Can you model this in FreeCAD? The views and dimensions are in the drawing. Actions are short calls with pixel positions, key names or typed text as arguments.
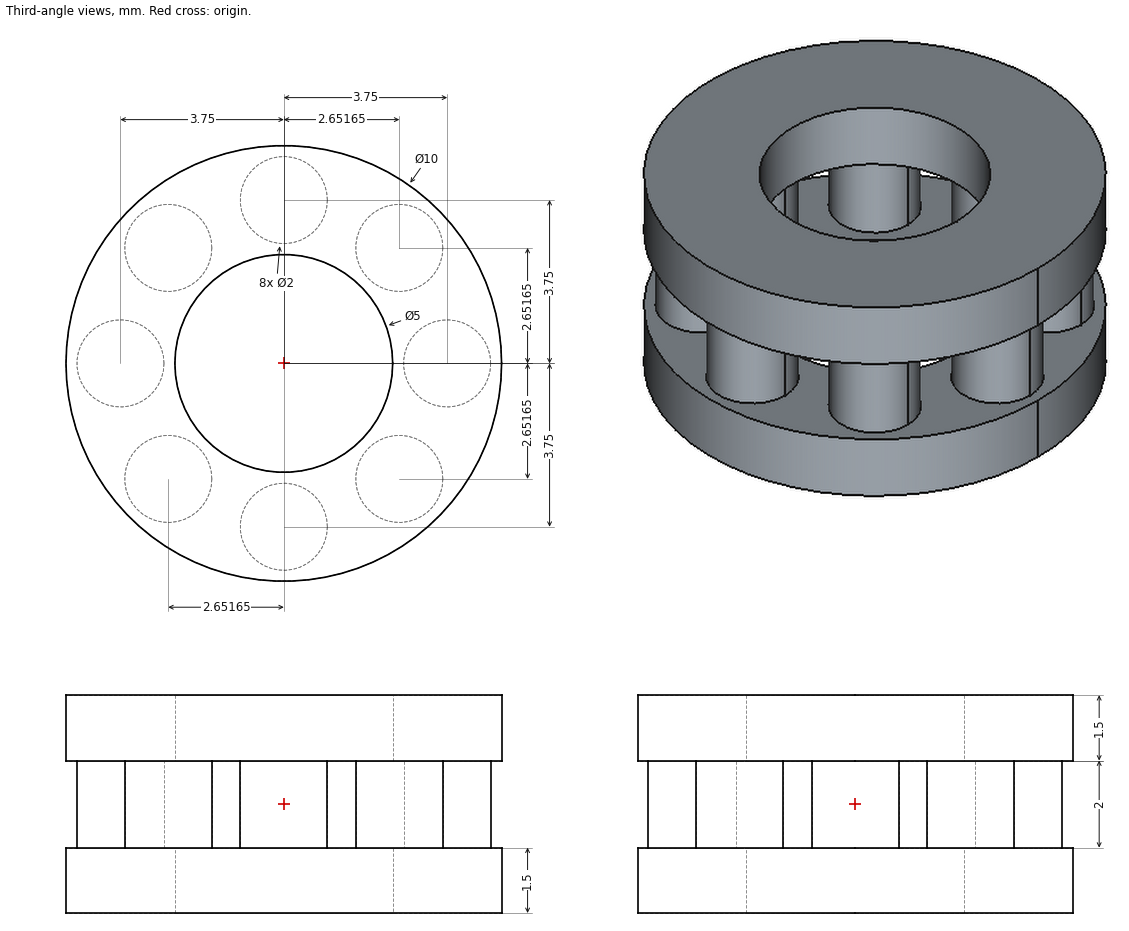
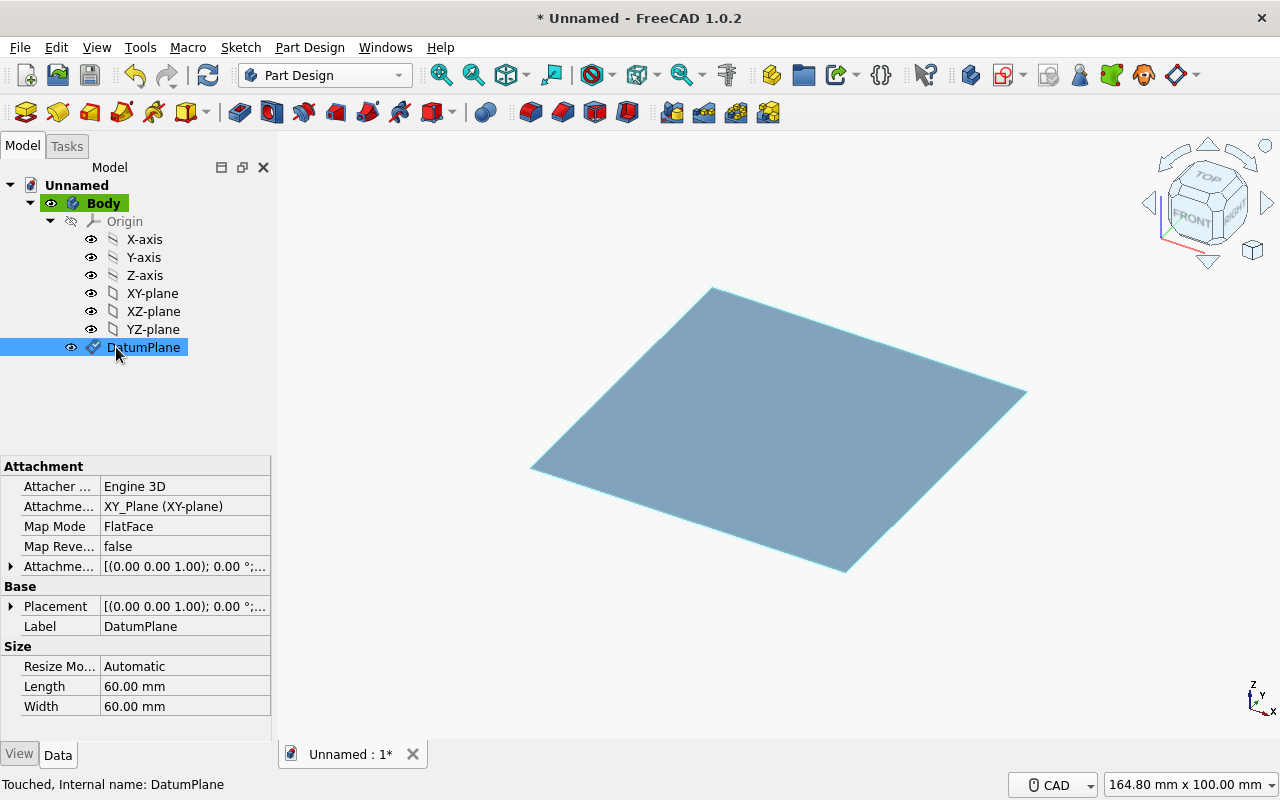
click(1004, 76)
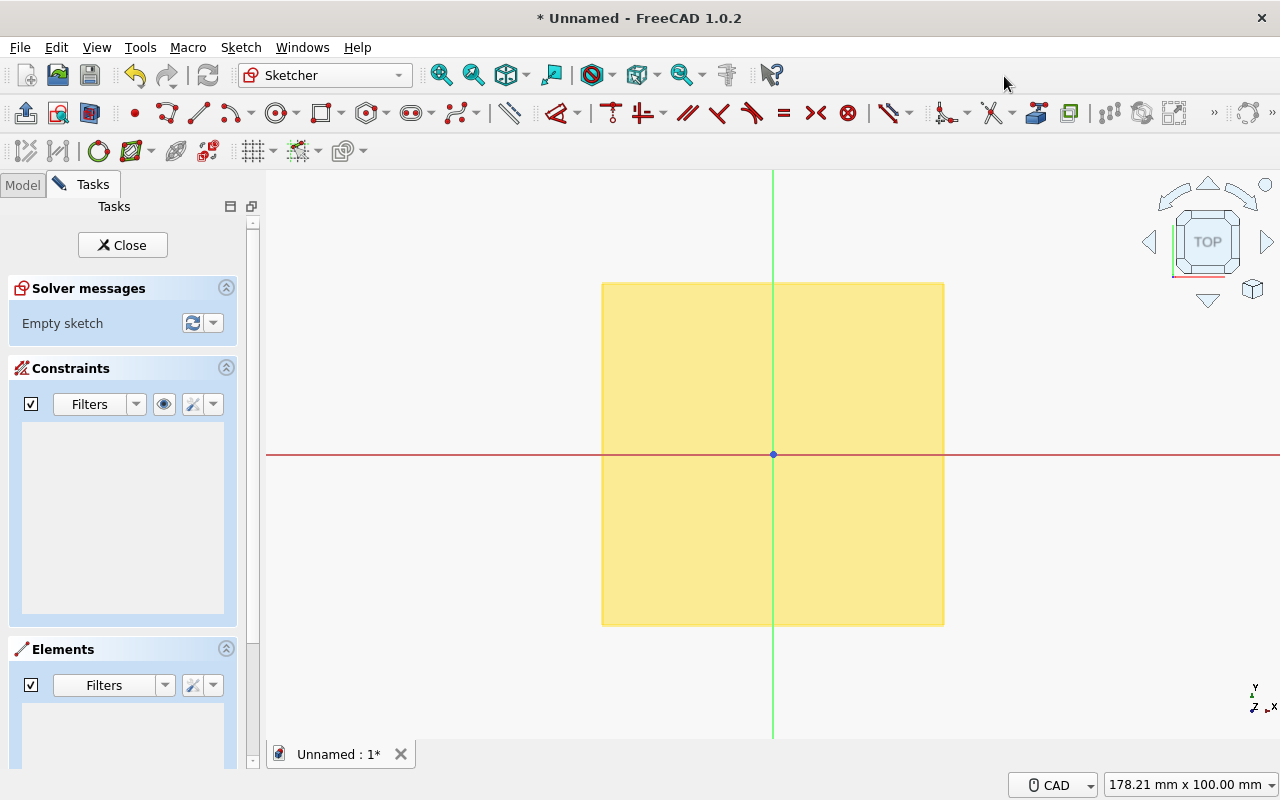
scroll(787, 455, up, 9)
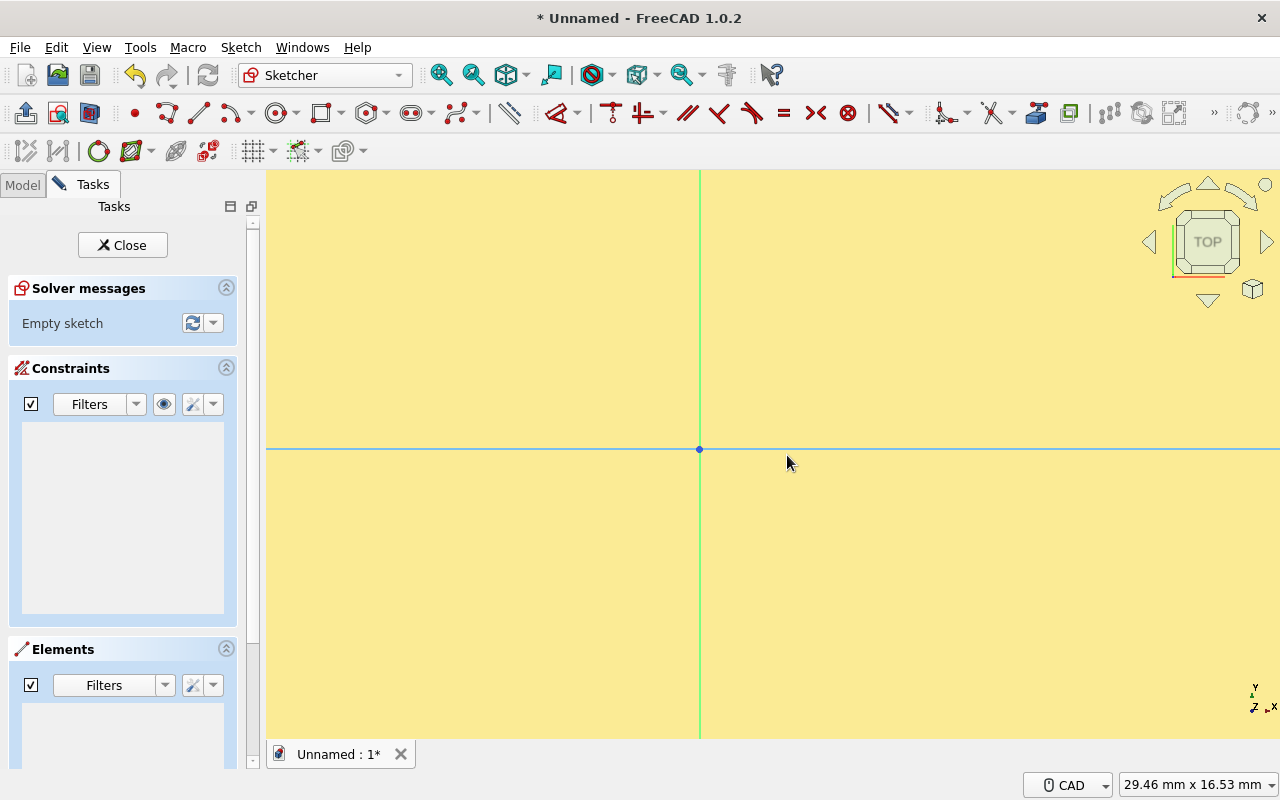
click(276, 114)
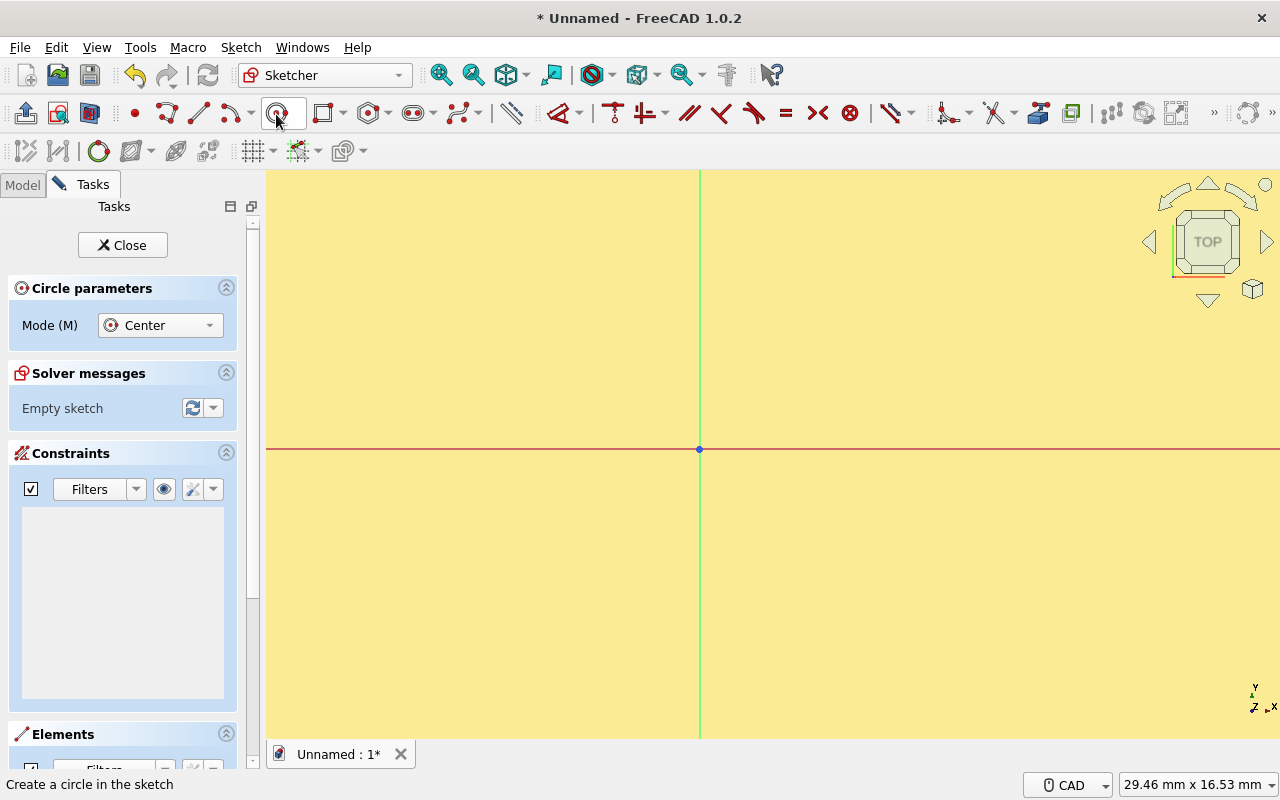
click(700, 449)
move(821, 328)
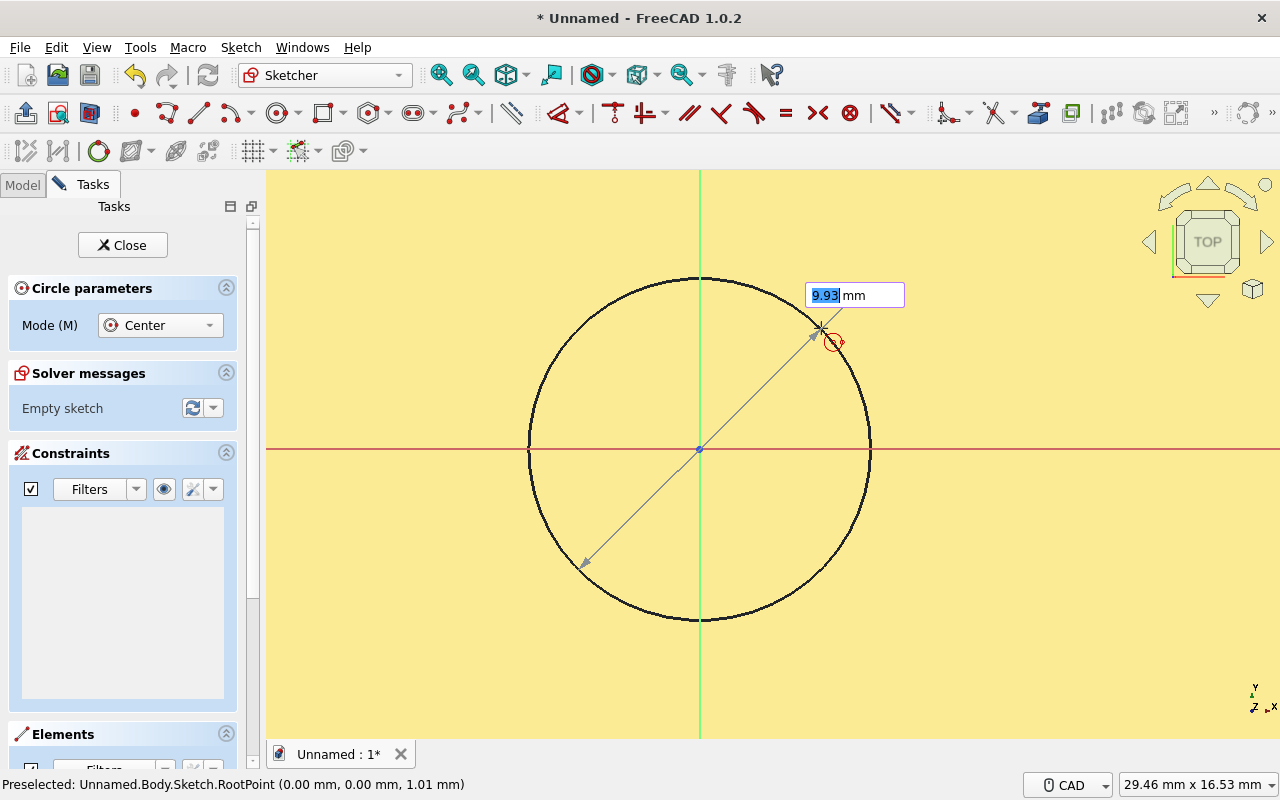
text(10)
key(Return)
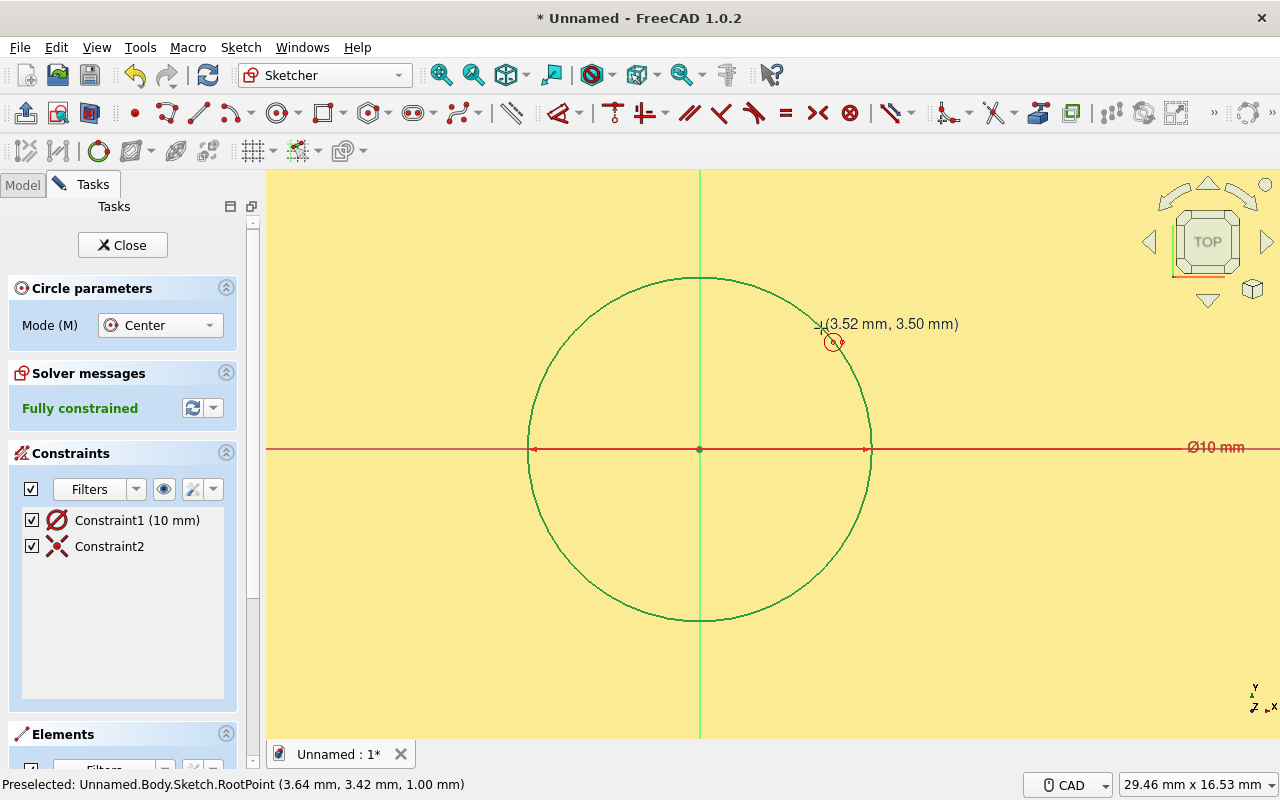
click(700, 449)
move(761, 389)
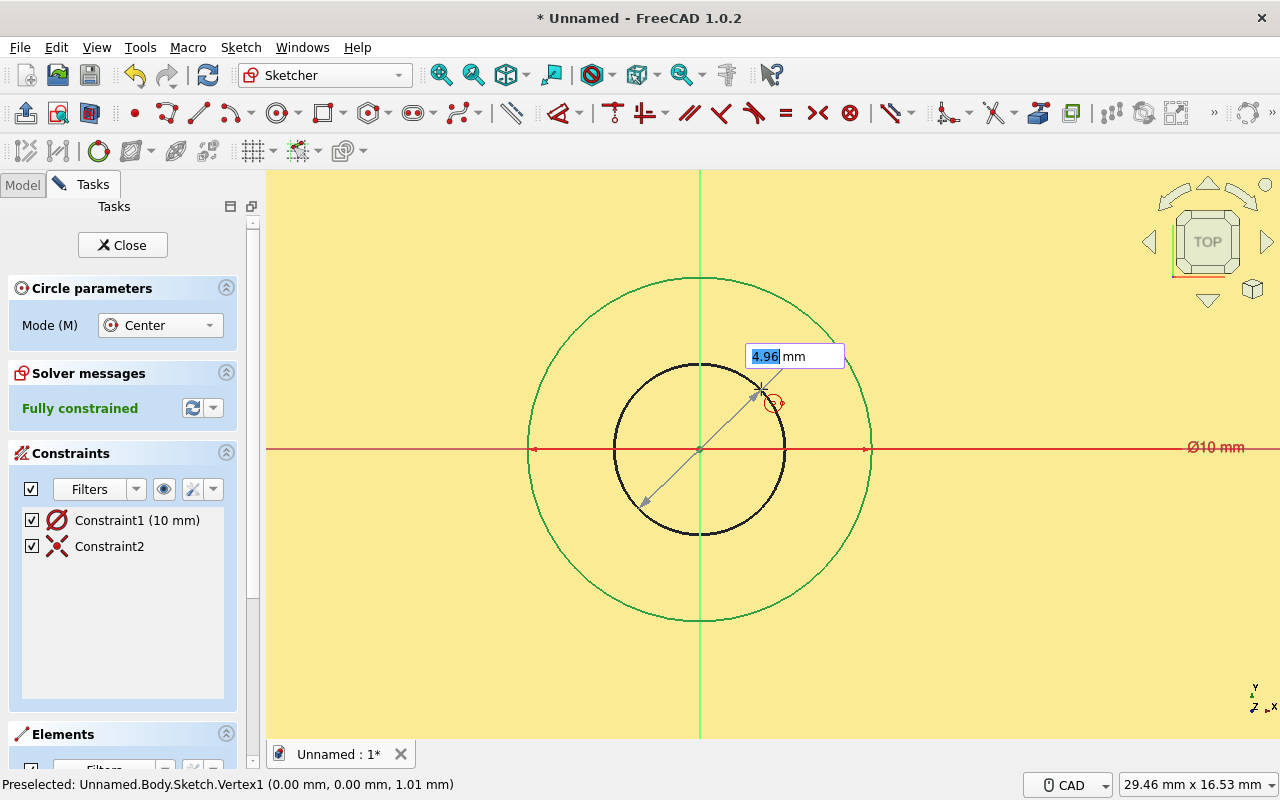
text(5)
key(Return)
key(Escape)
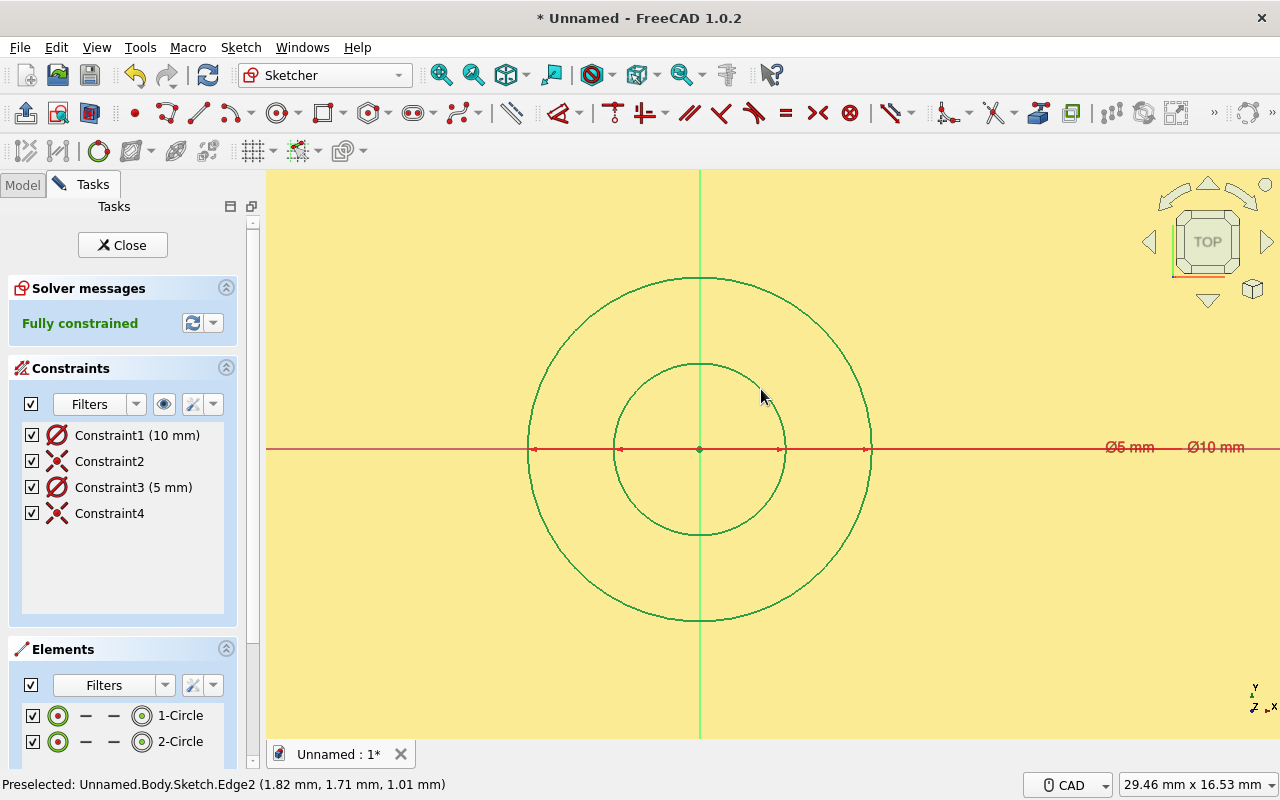
click(123, 245)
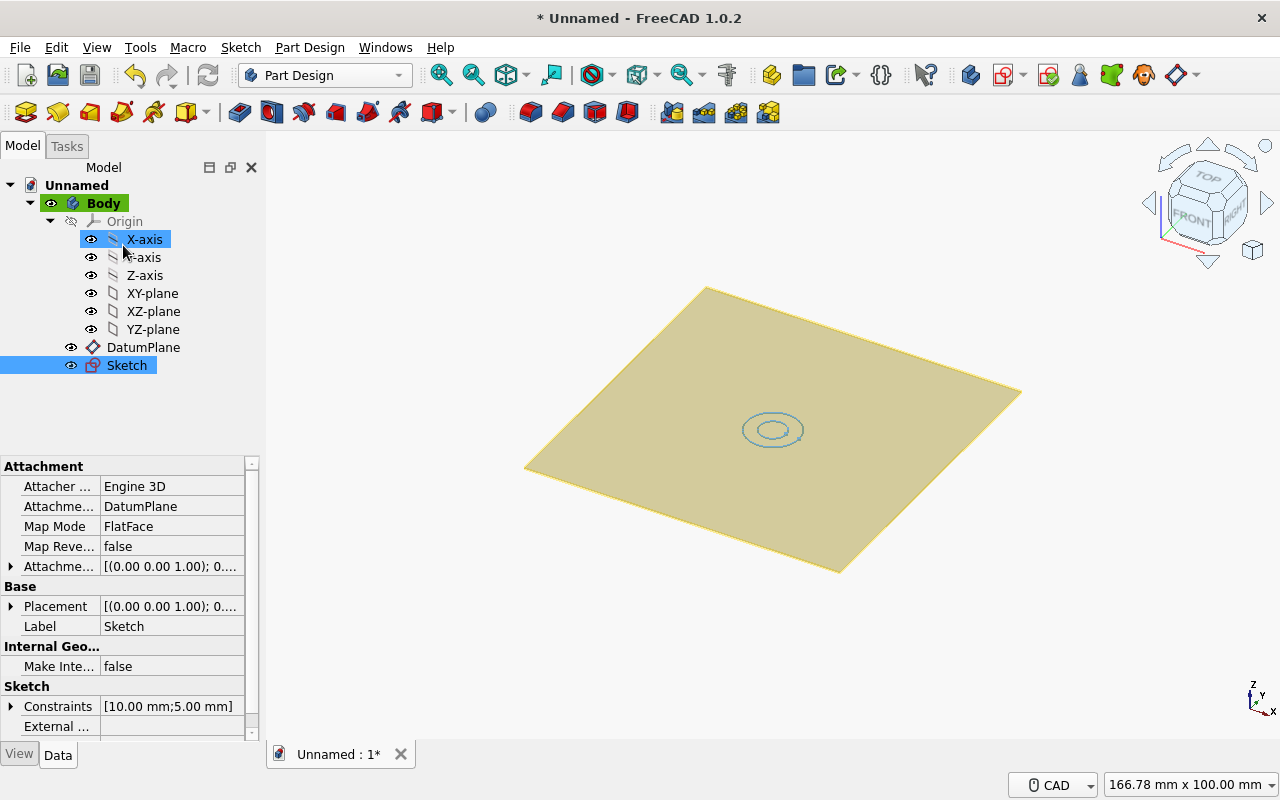
click(26, 112)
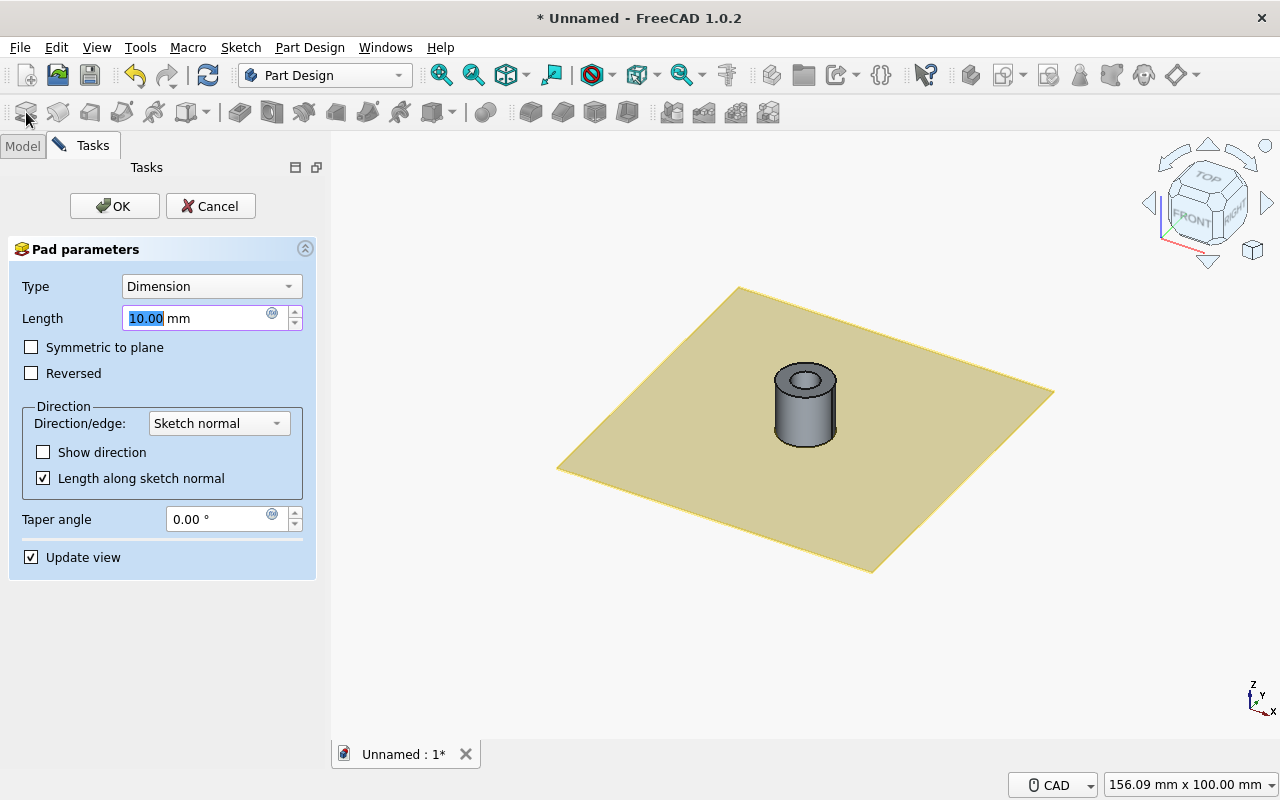
text(1.5)
key(Tab)